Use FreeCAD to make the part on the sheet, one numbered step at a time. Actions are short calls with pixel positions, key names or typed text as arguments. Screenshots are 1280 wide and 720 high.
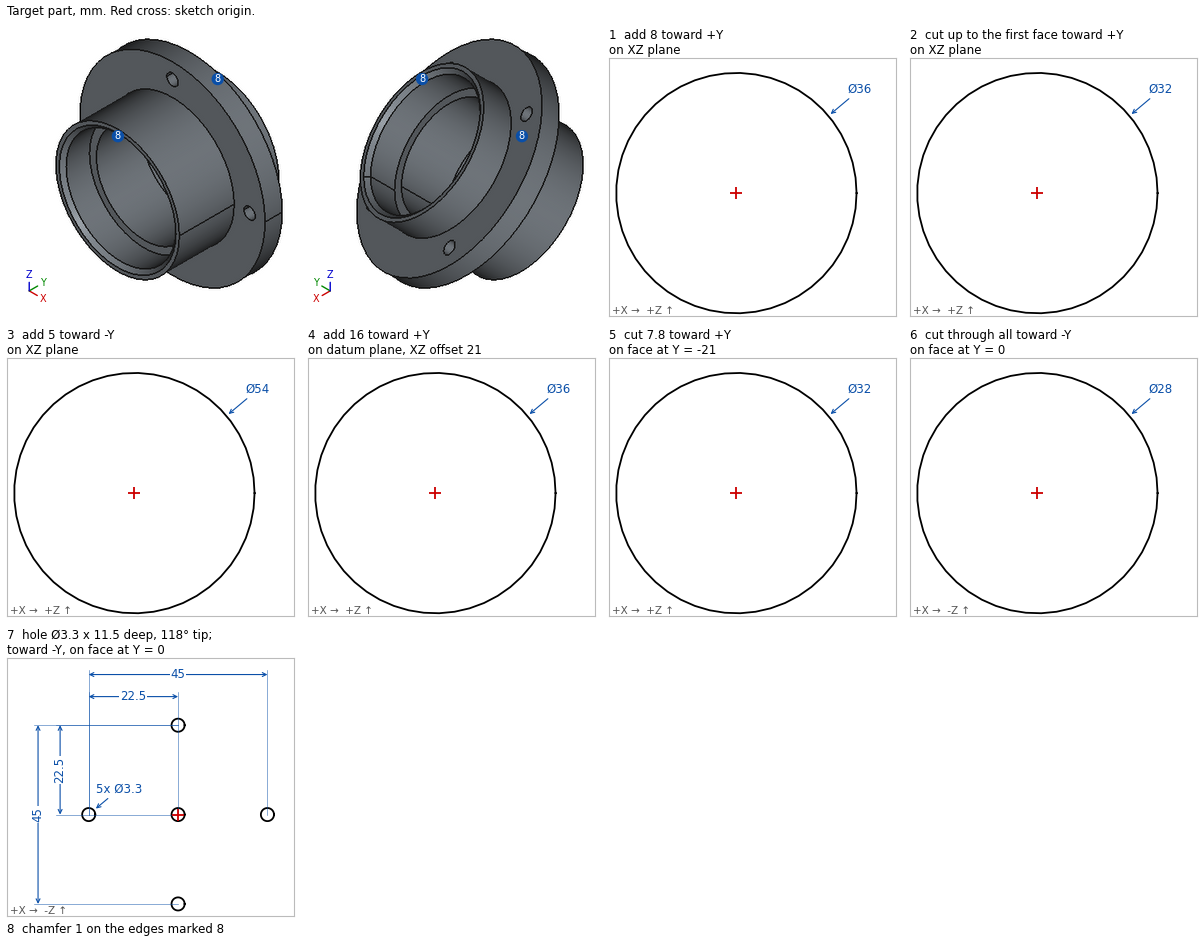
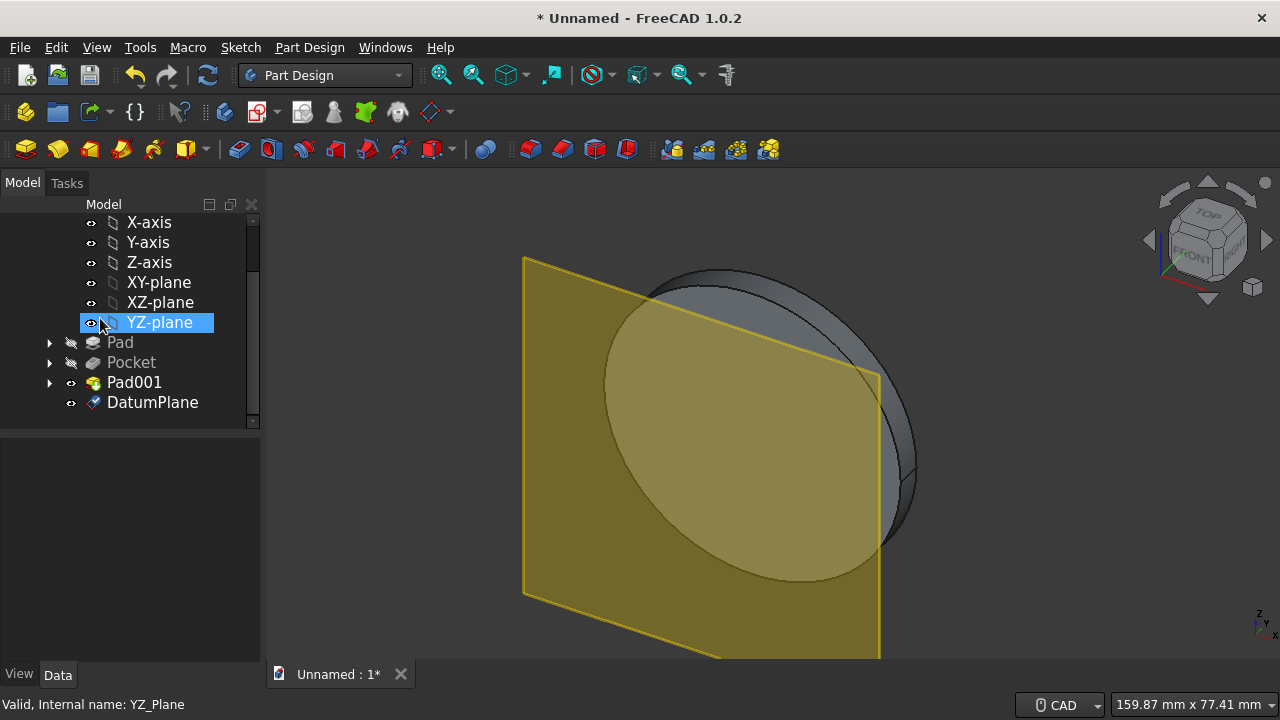
click(116, 403)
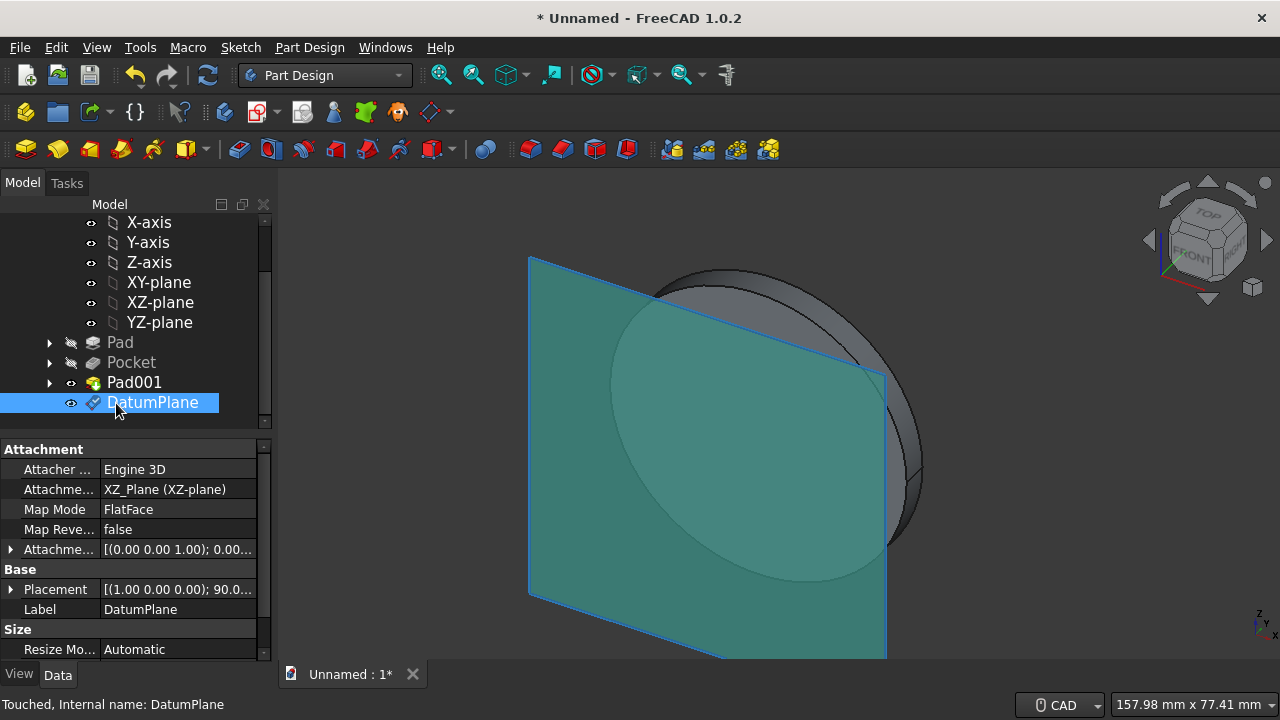
click(258, 112)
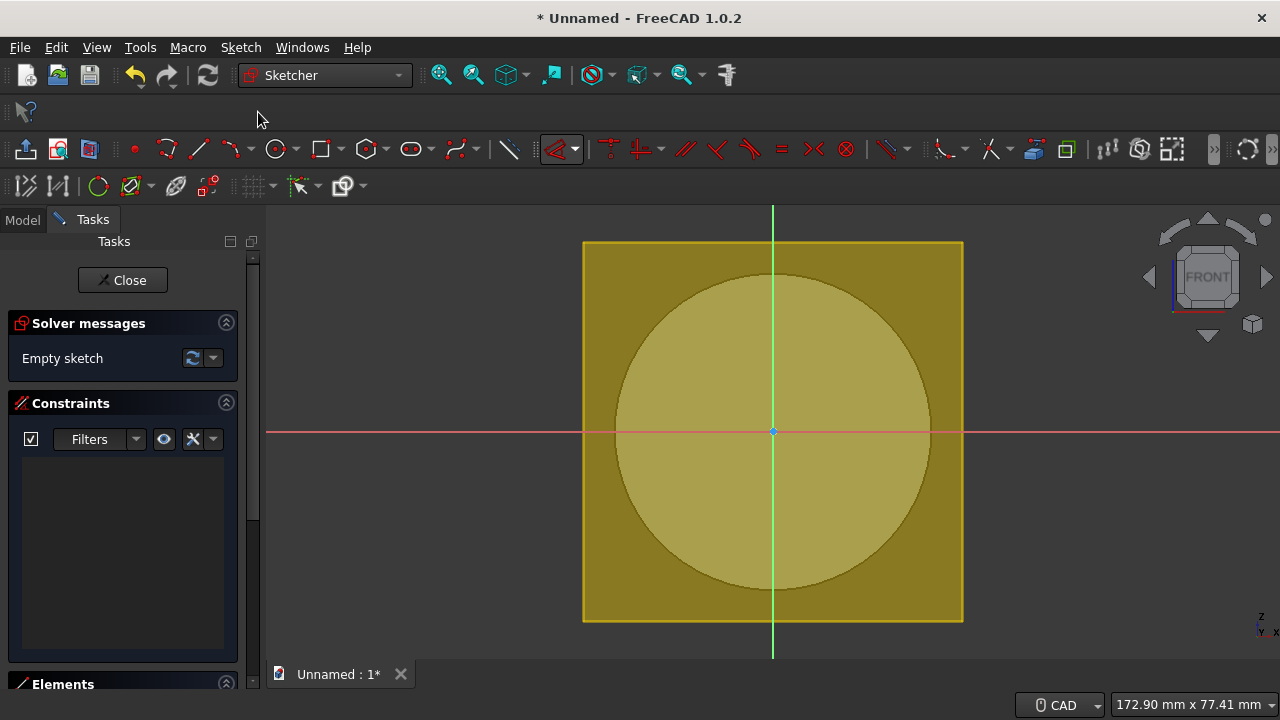
click(276, 150)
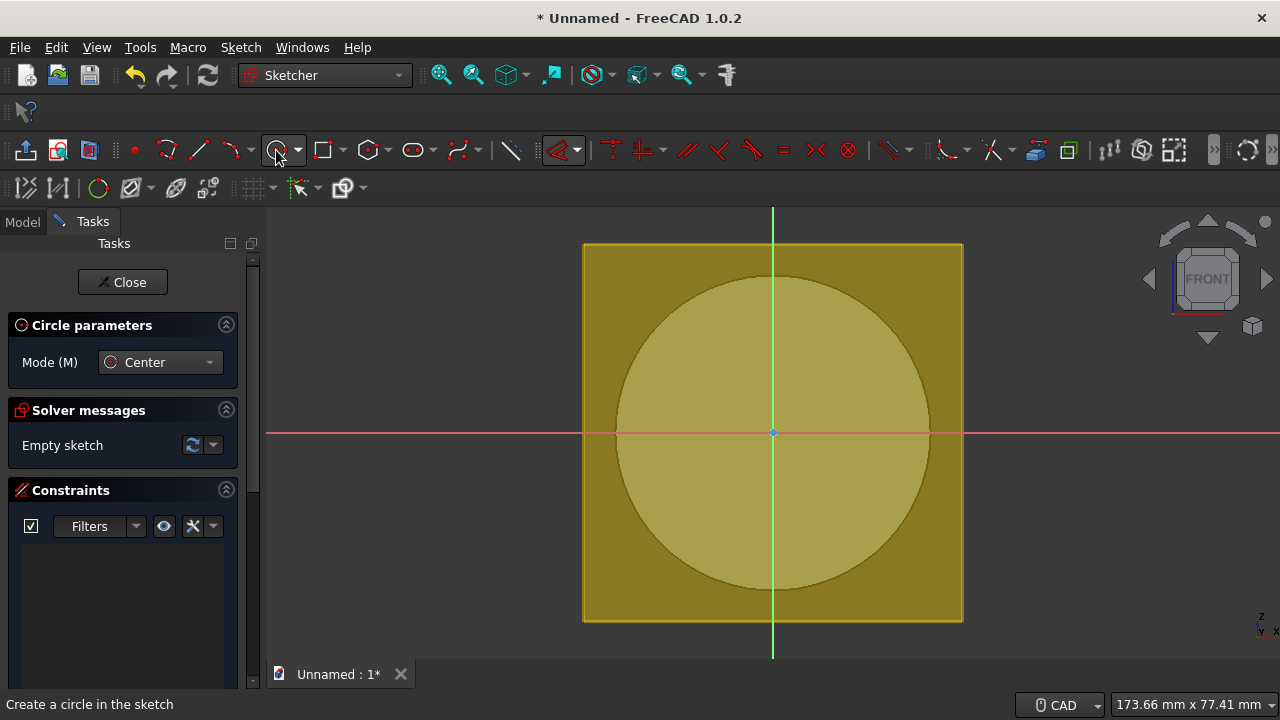
click(773, 433)
click(847, 359)
key(Escape)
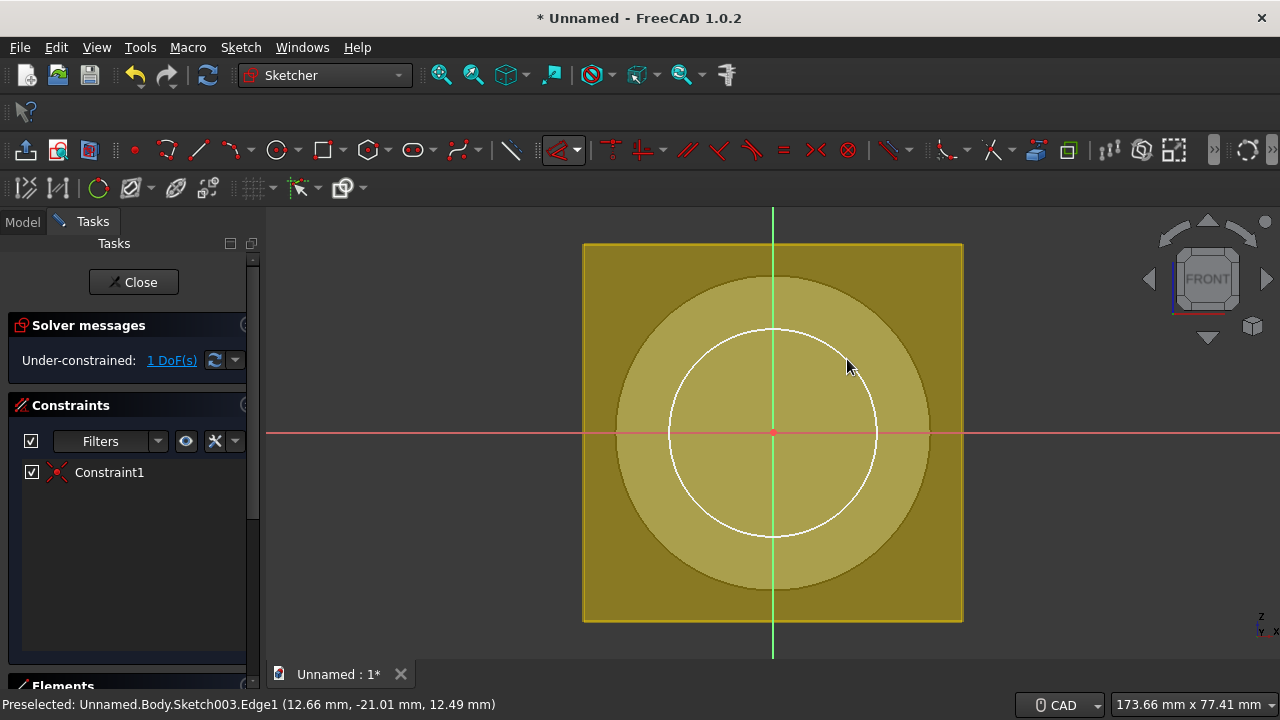
click(846, 359)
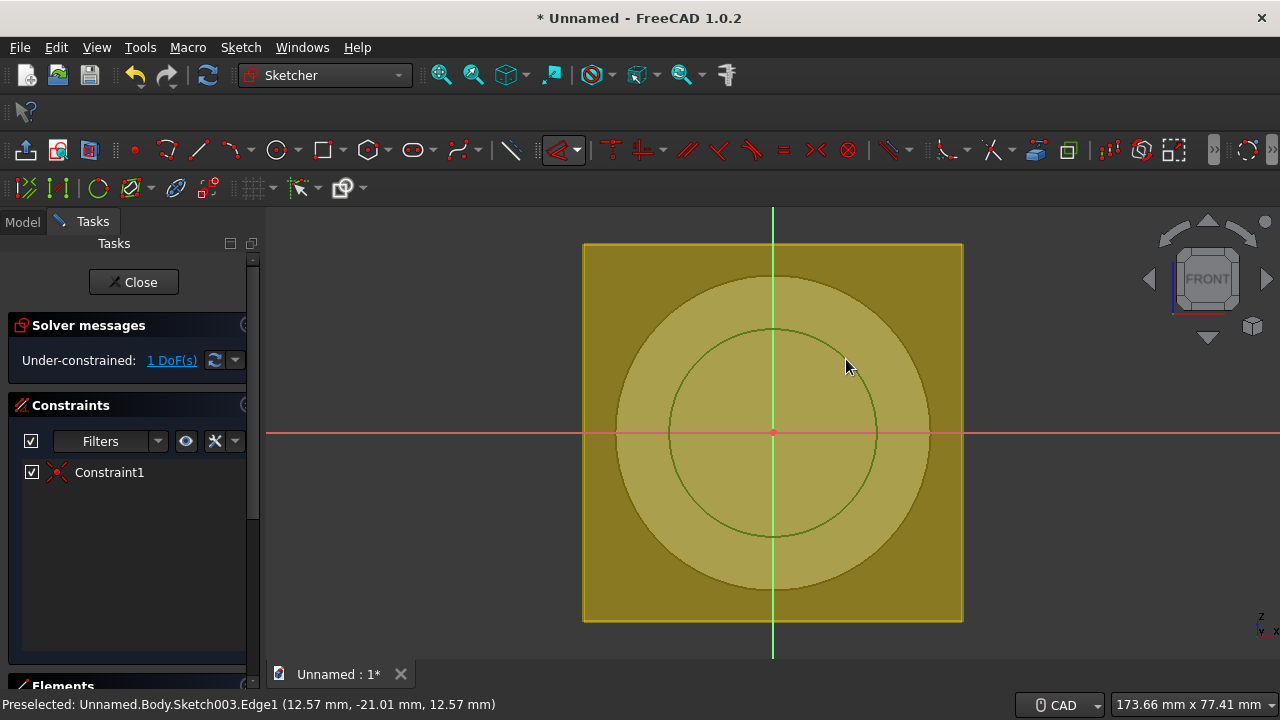
key(k)
key(o)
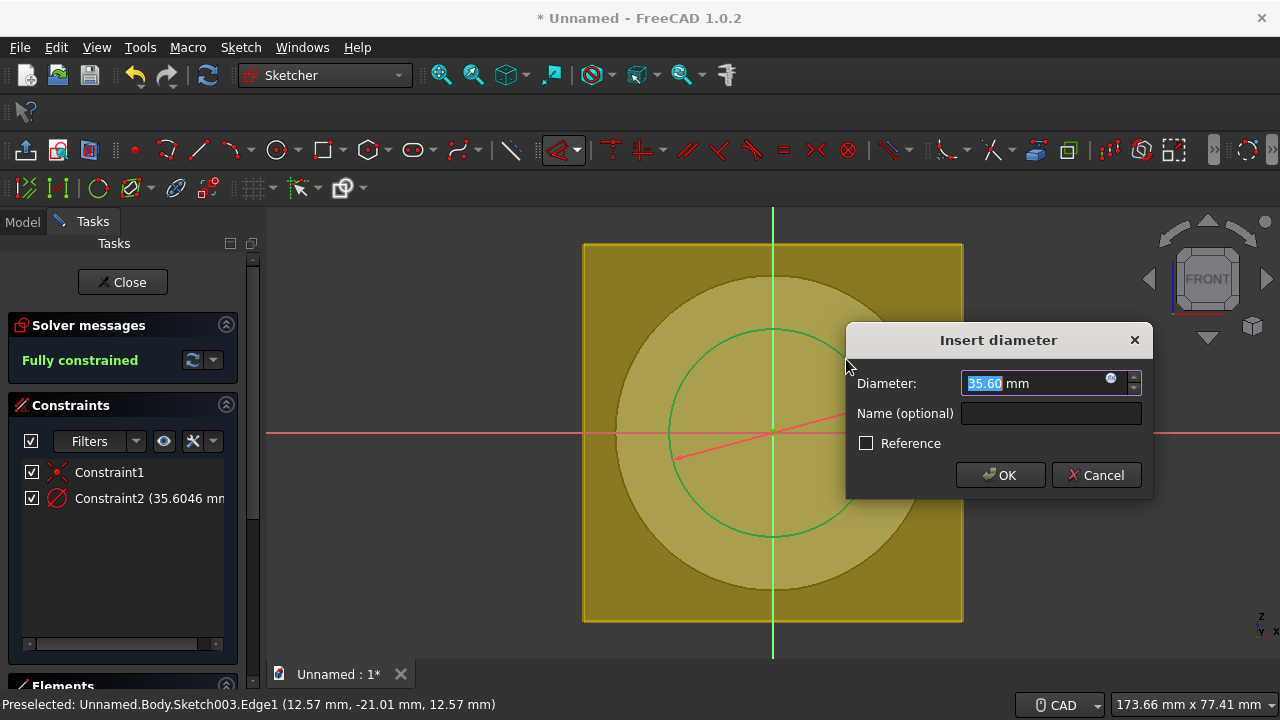
text(36)
key(Return)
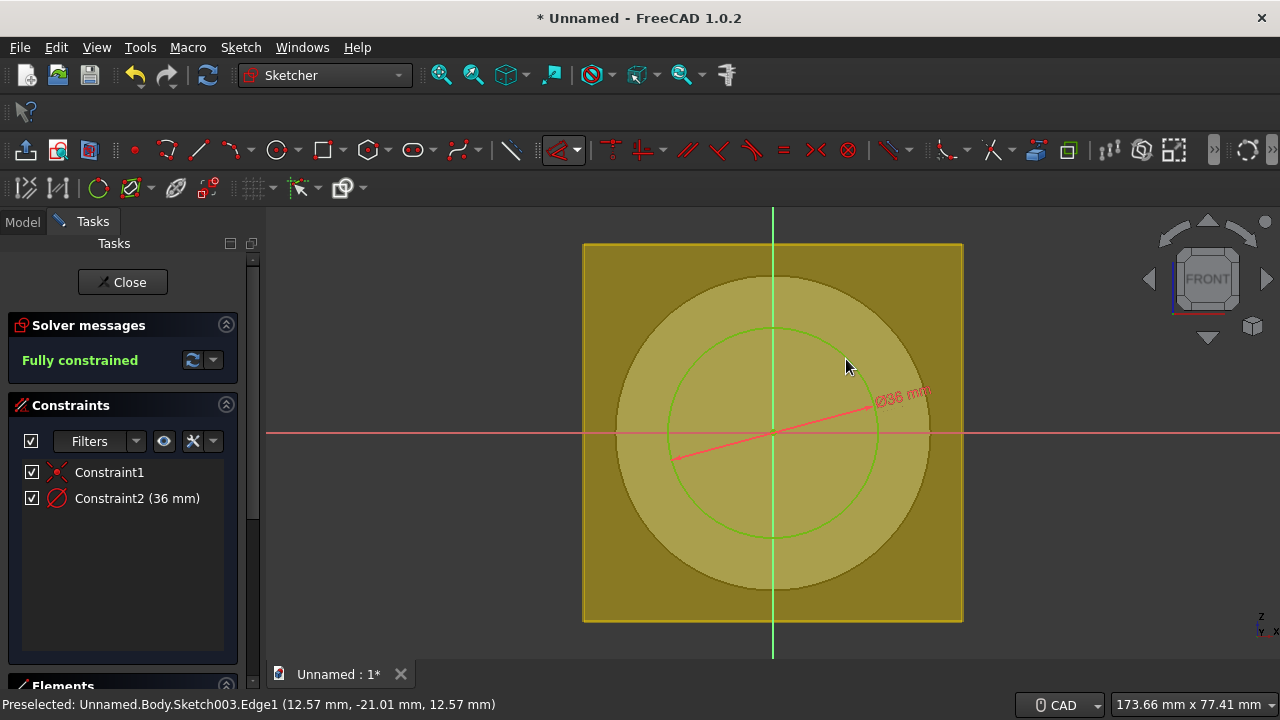
click(123, 282)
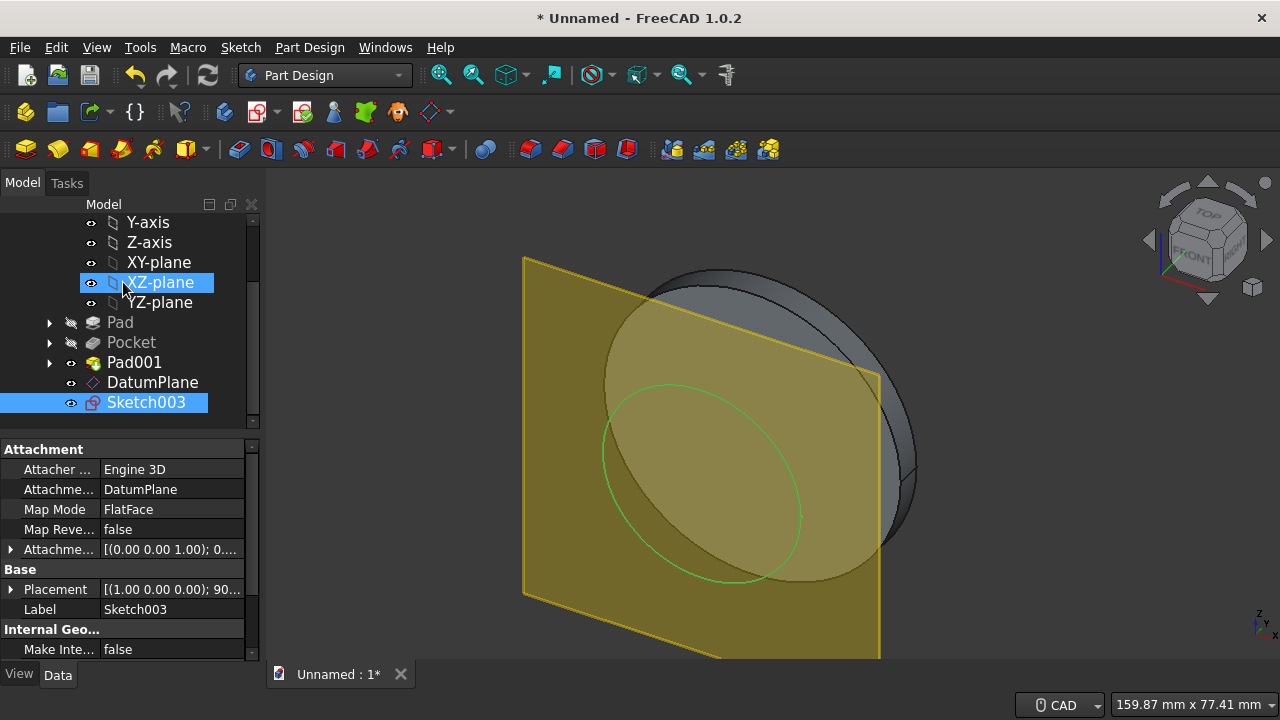
click(26, 150)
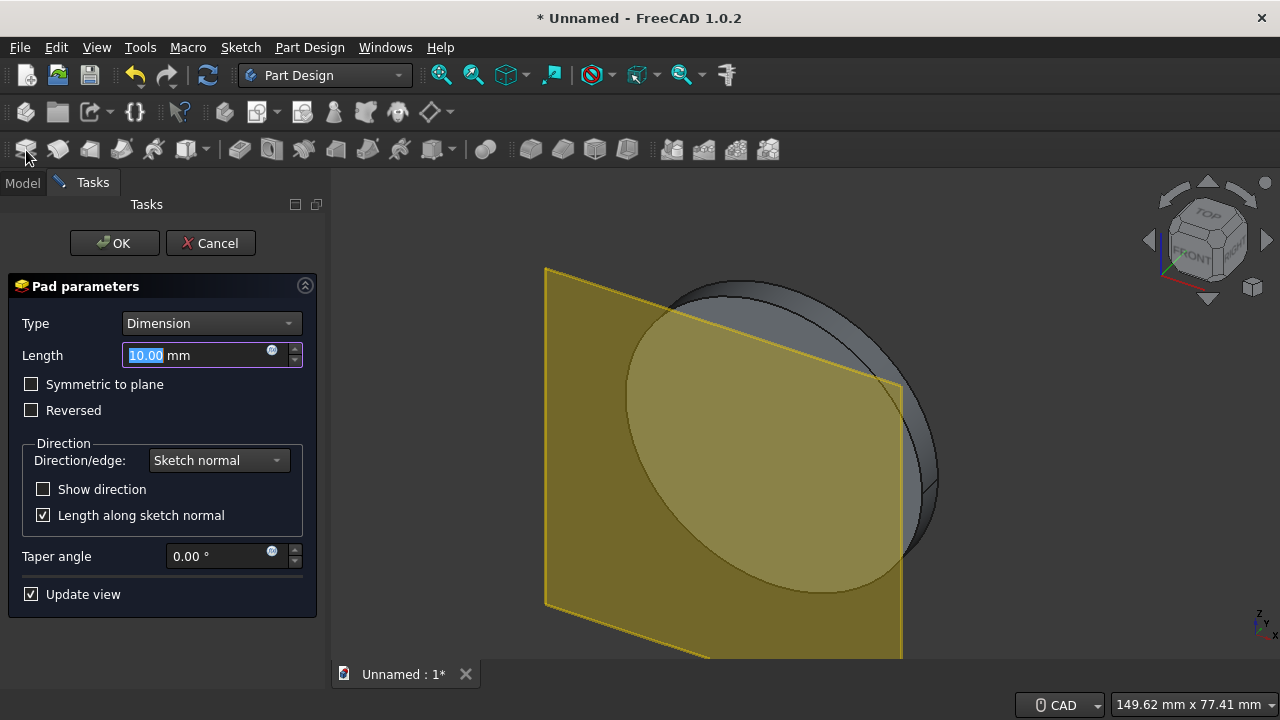
text(16)
key(Tab)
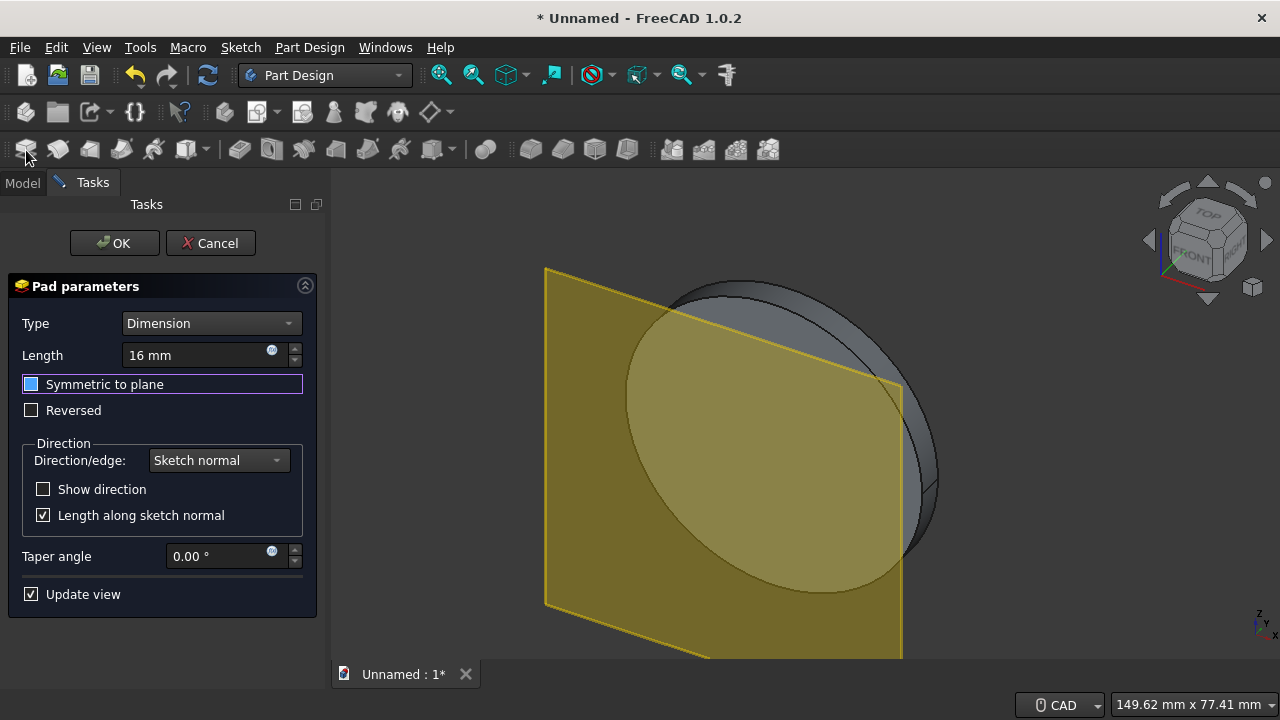
click(30, 410)